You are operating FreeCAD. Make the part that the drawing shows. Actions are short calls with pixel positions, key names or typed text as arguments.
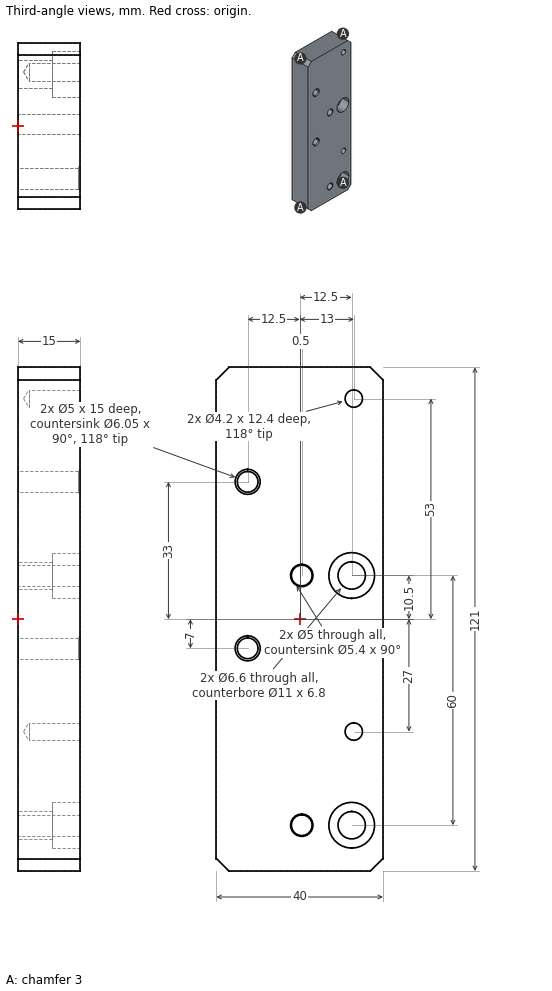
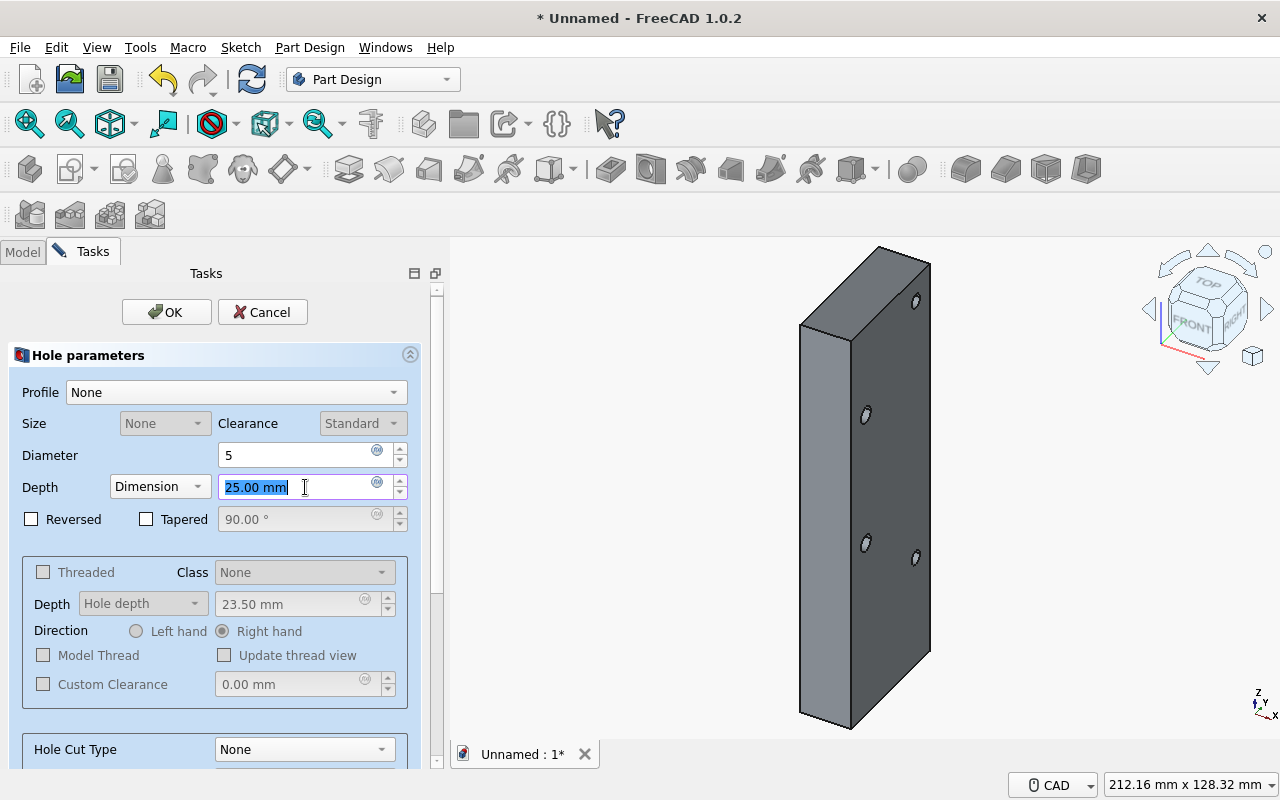
text(15)
key(Tab)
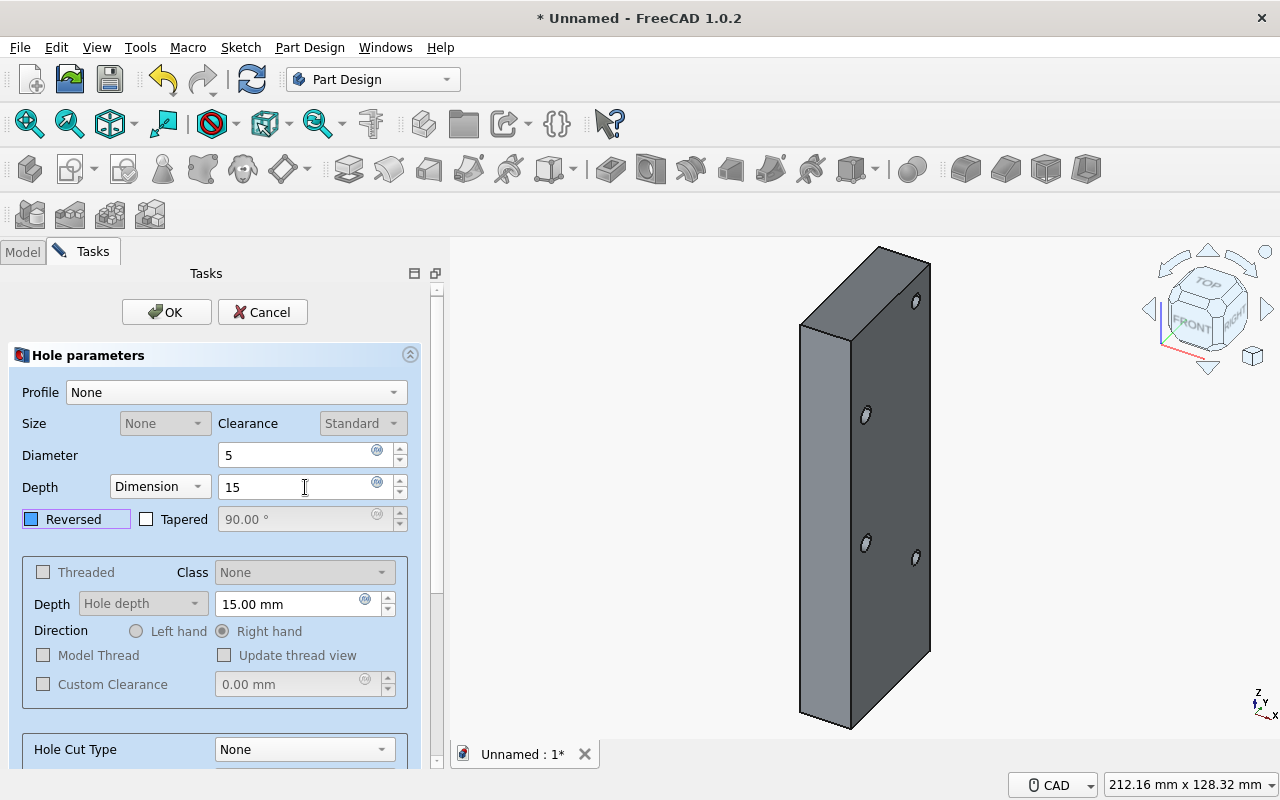
click(306, 750)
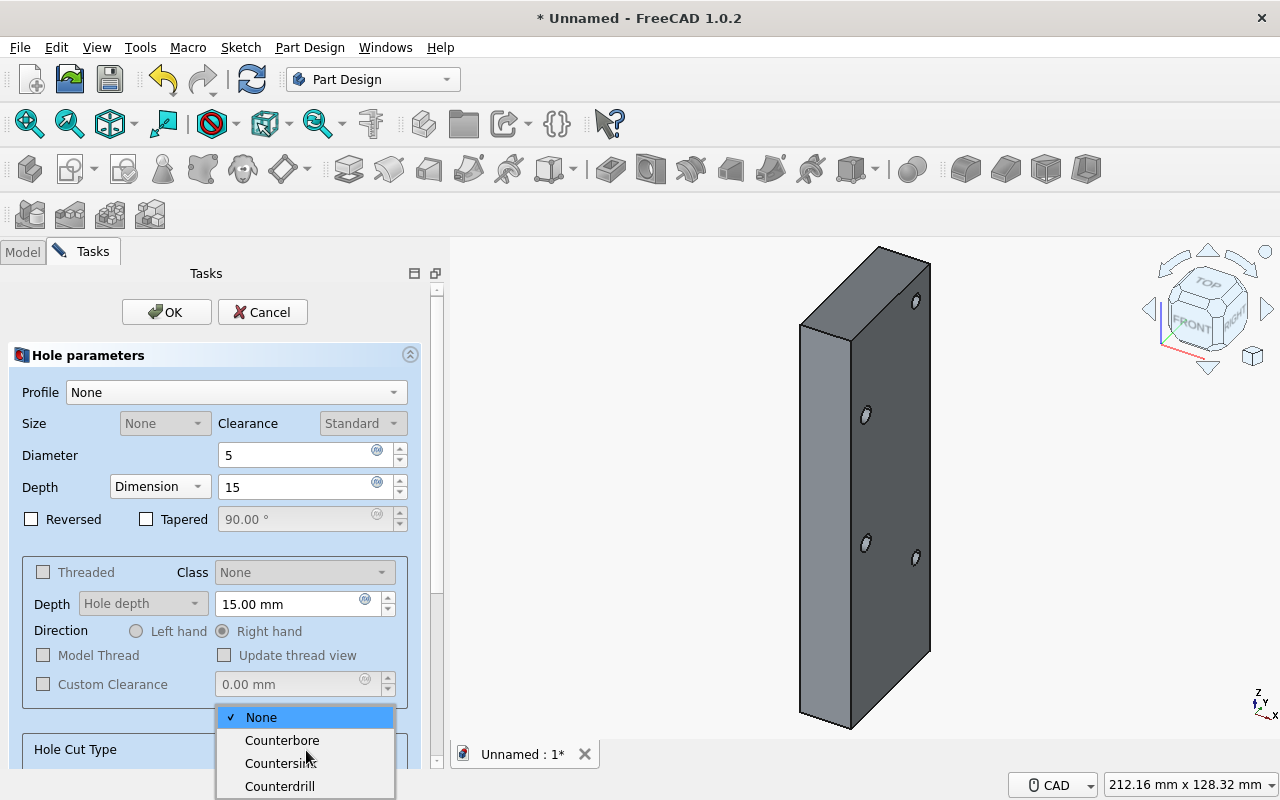
click(304, 764)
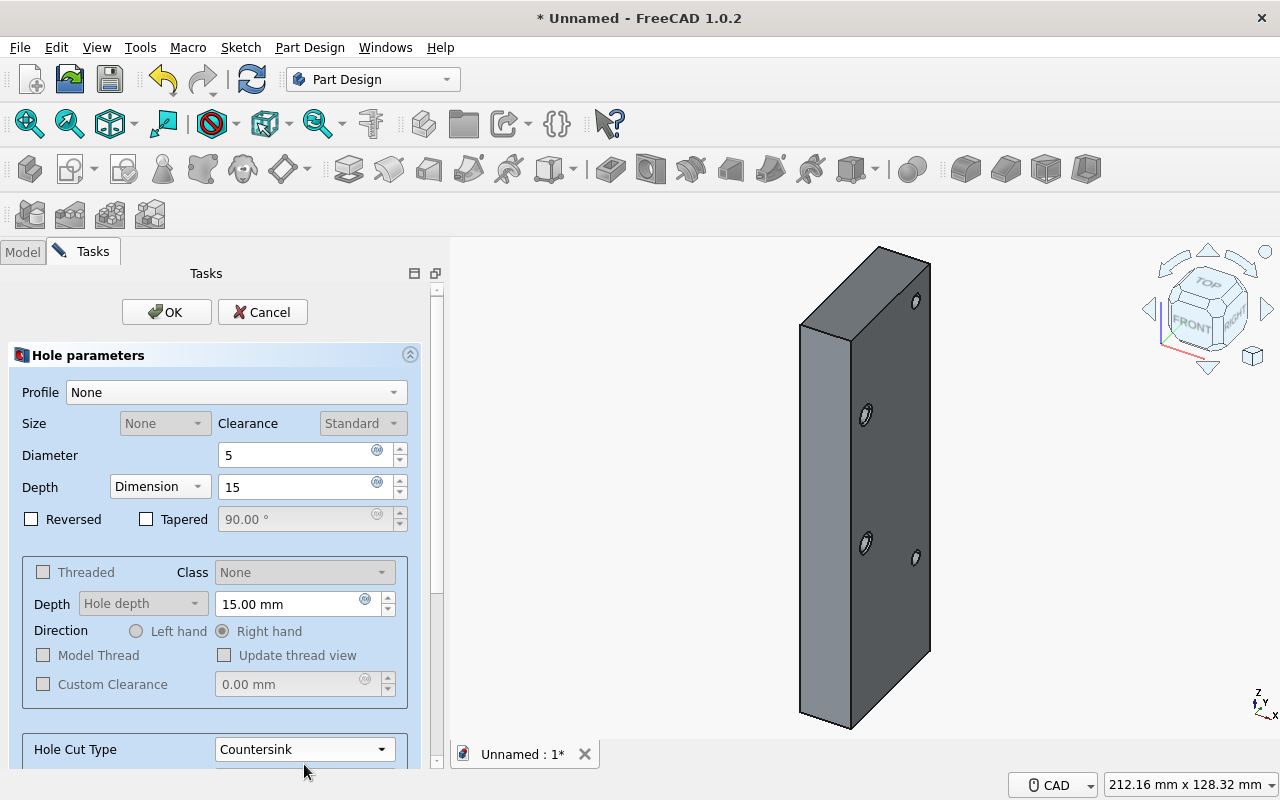
scroll(437, 526, down, 2)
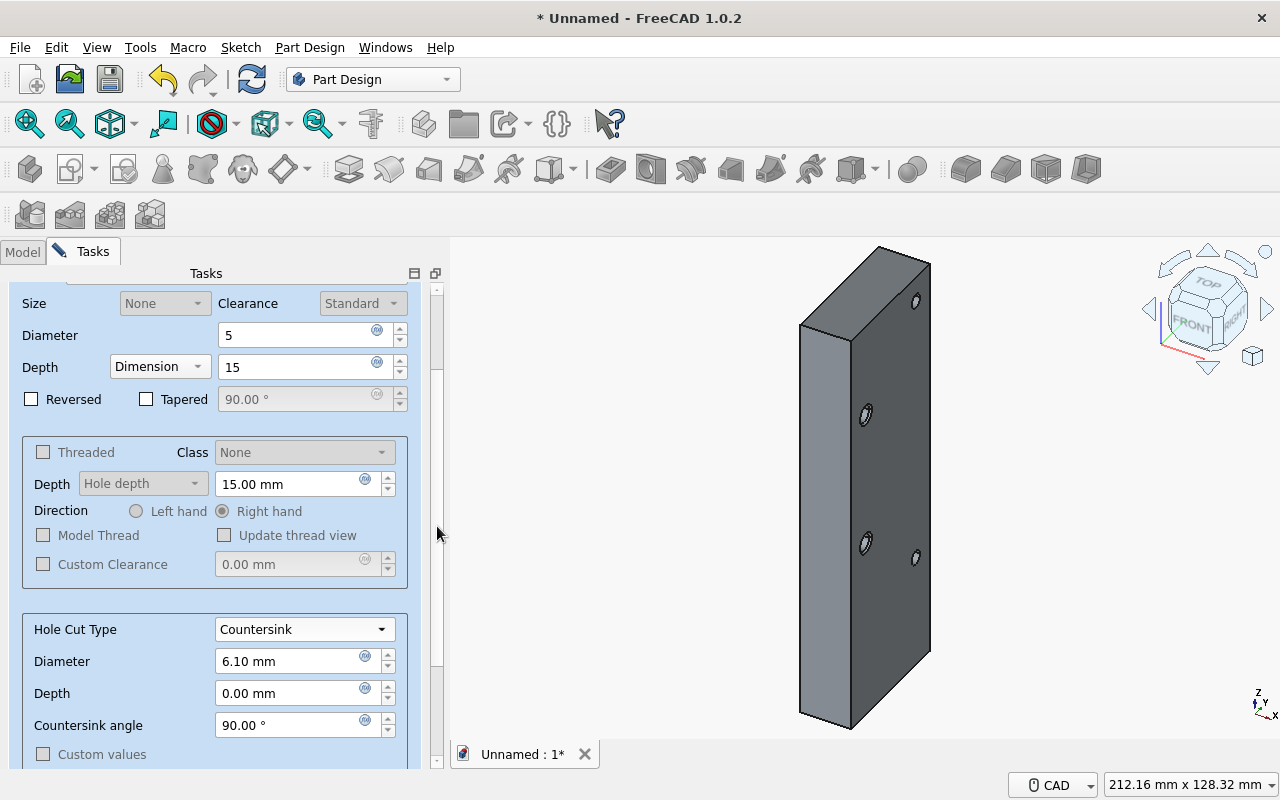
triple_click(298, 661)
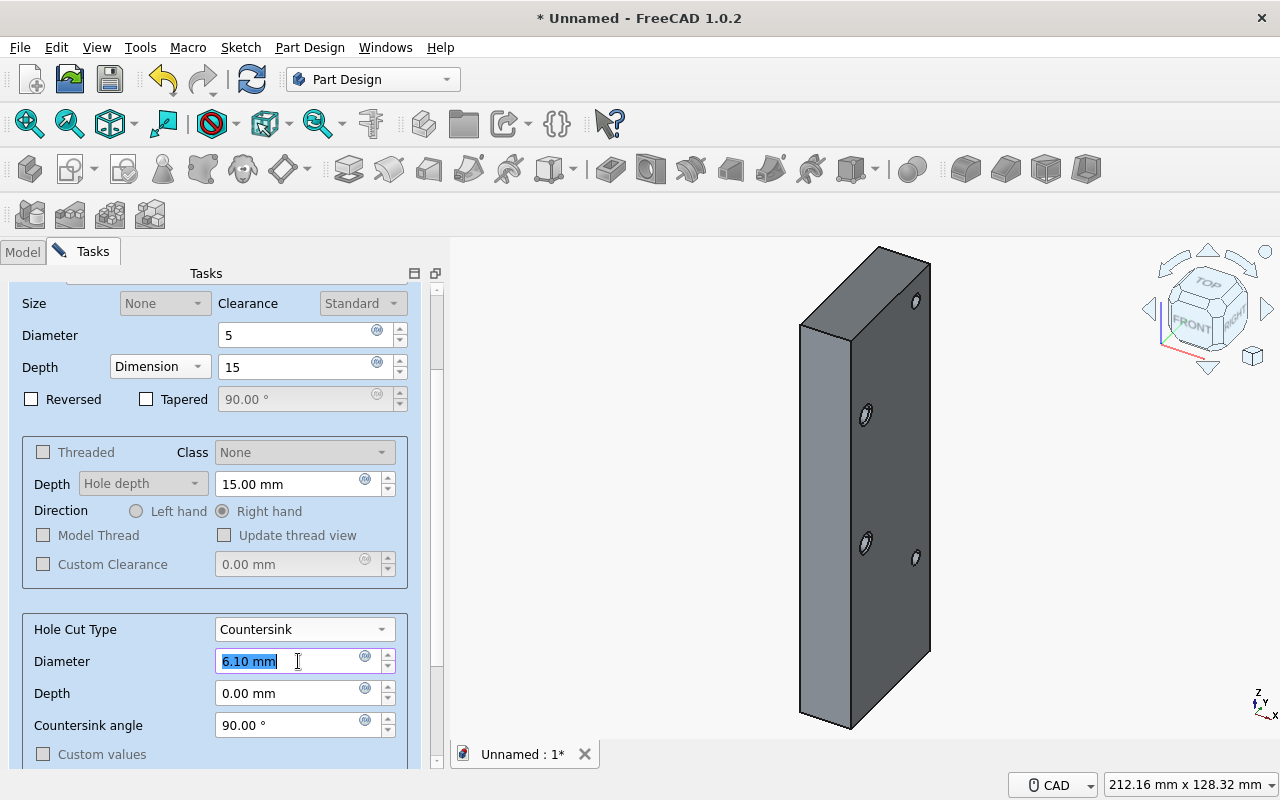
text(6.05)
key(Tab)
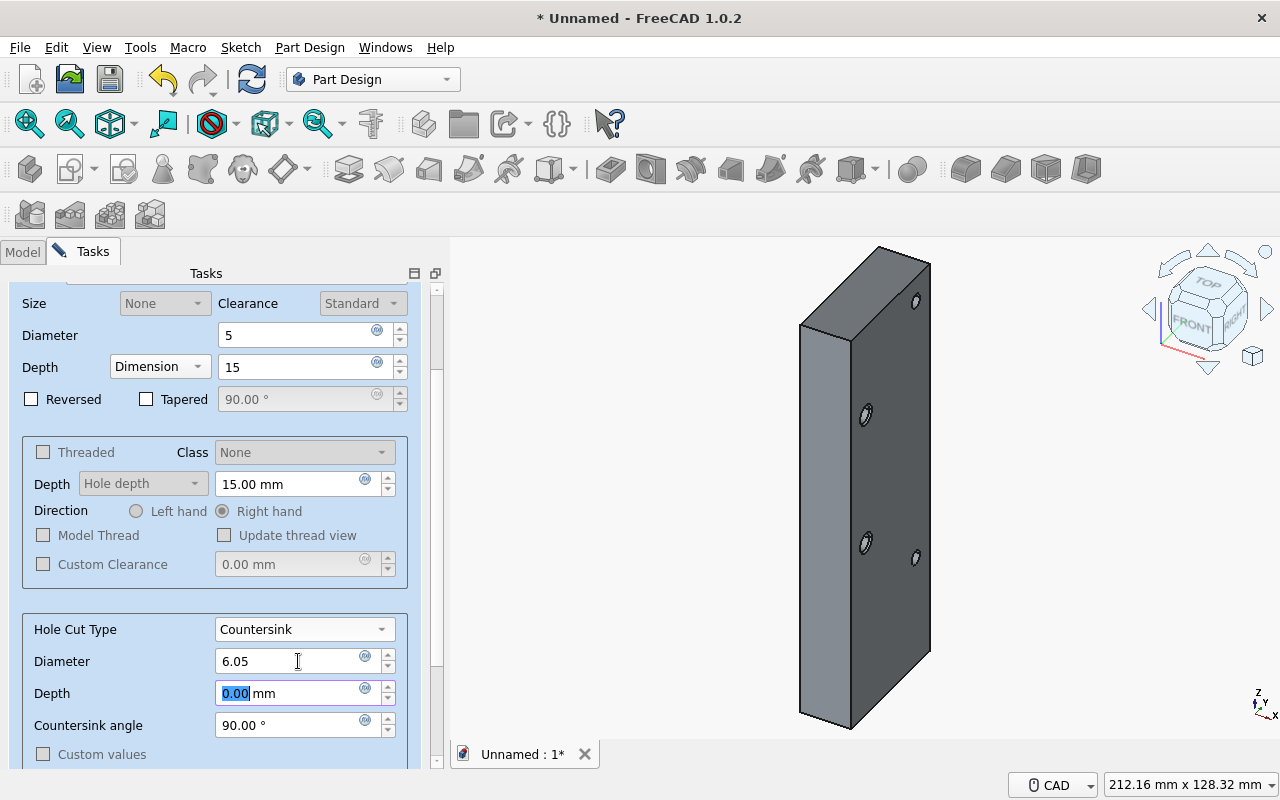
scroll(437, 526, up, 3)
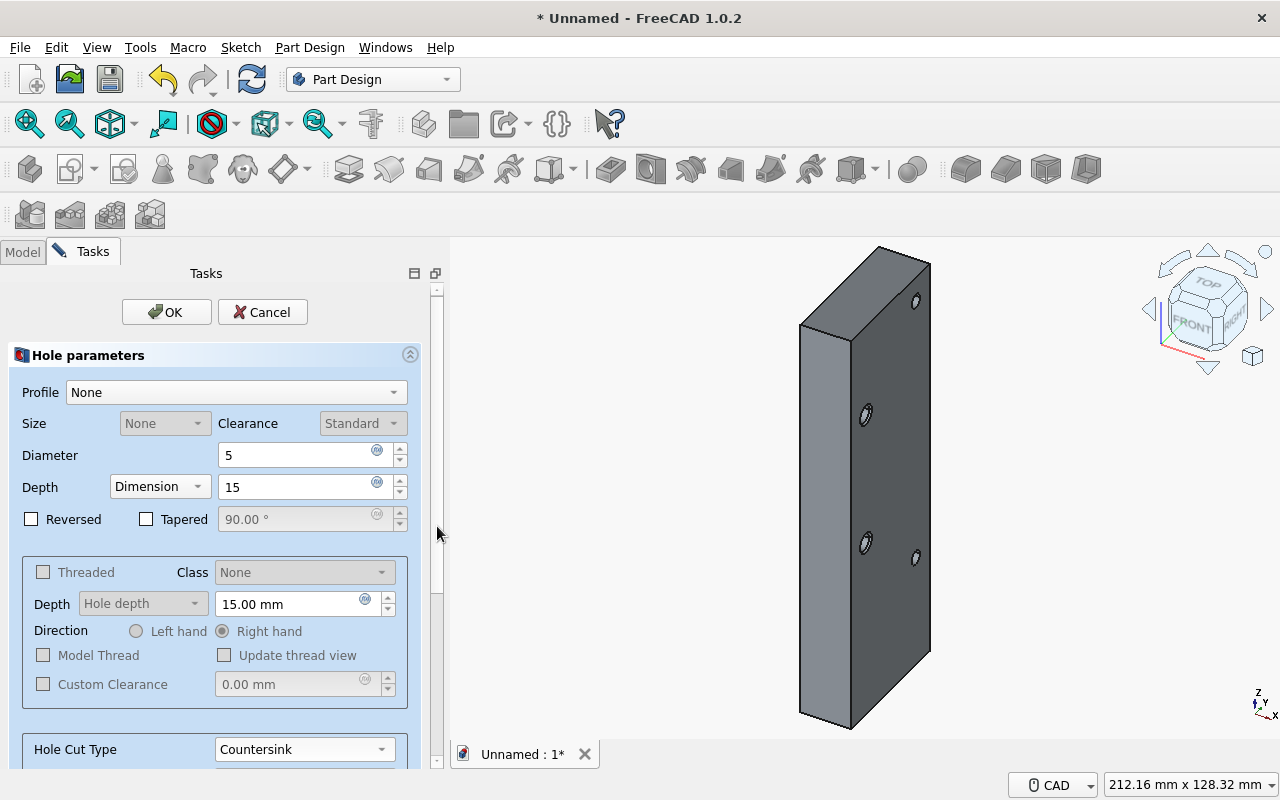
click(167, 312)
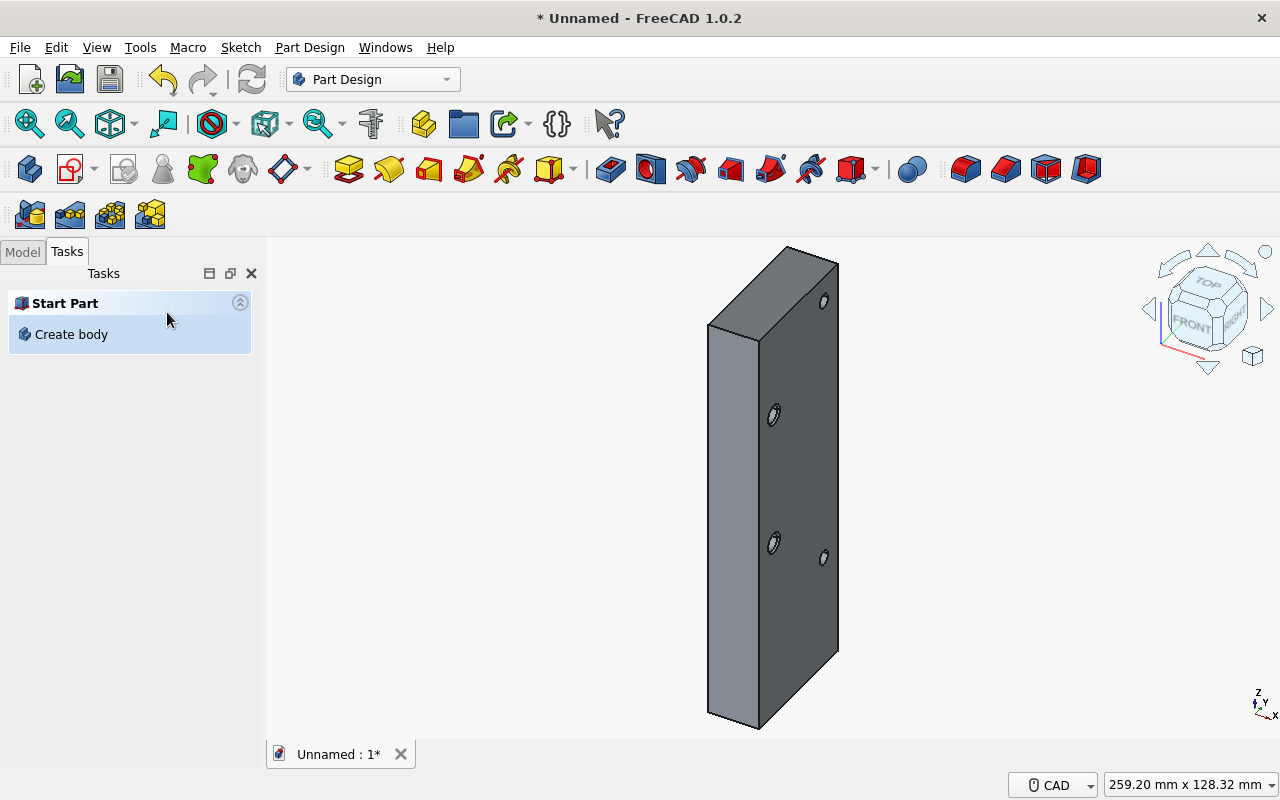
click(798, 440)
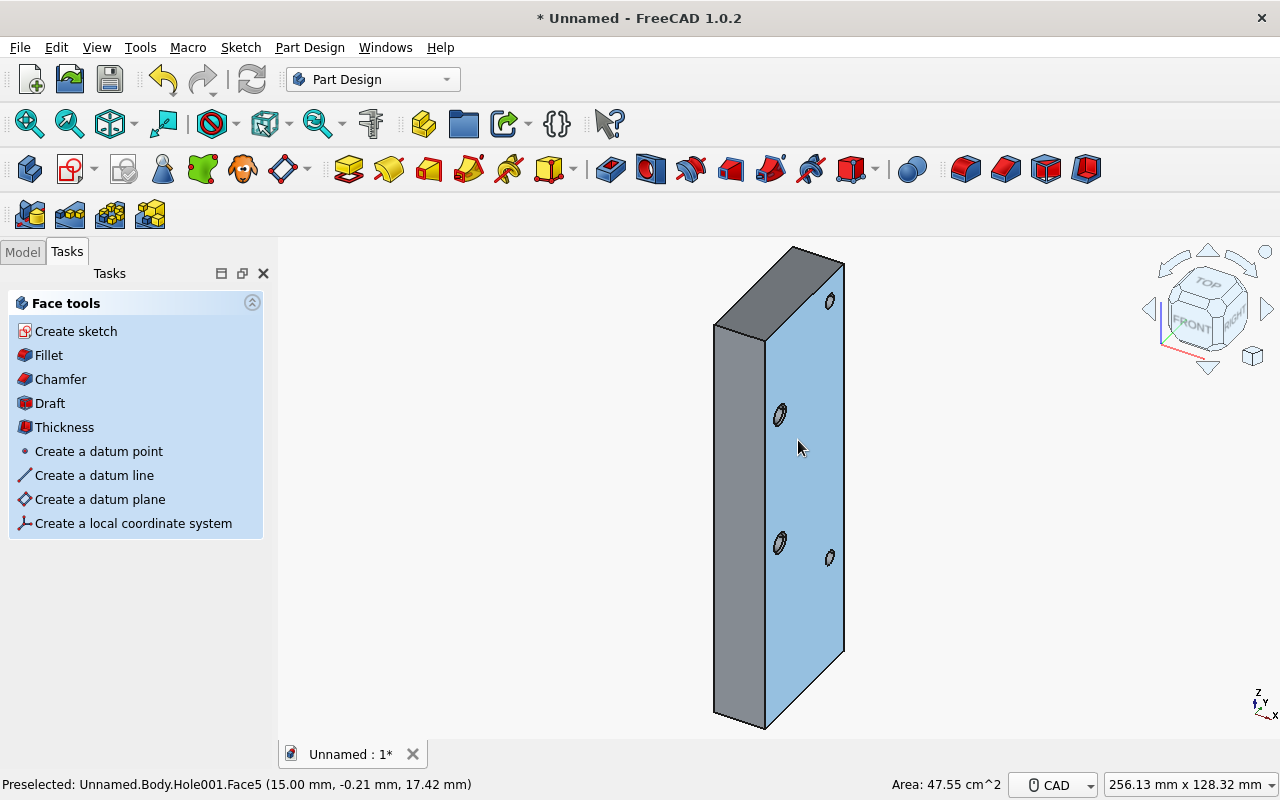
click(70, 170)